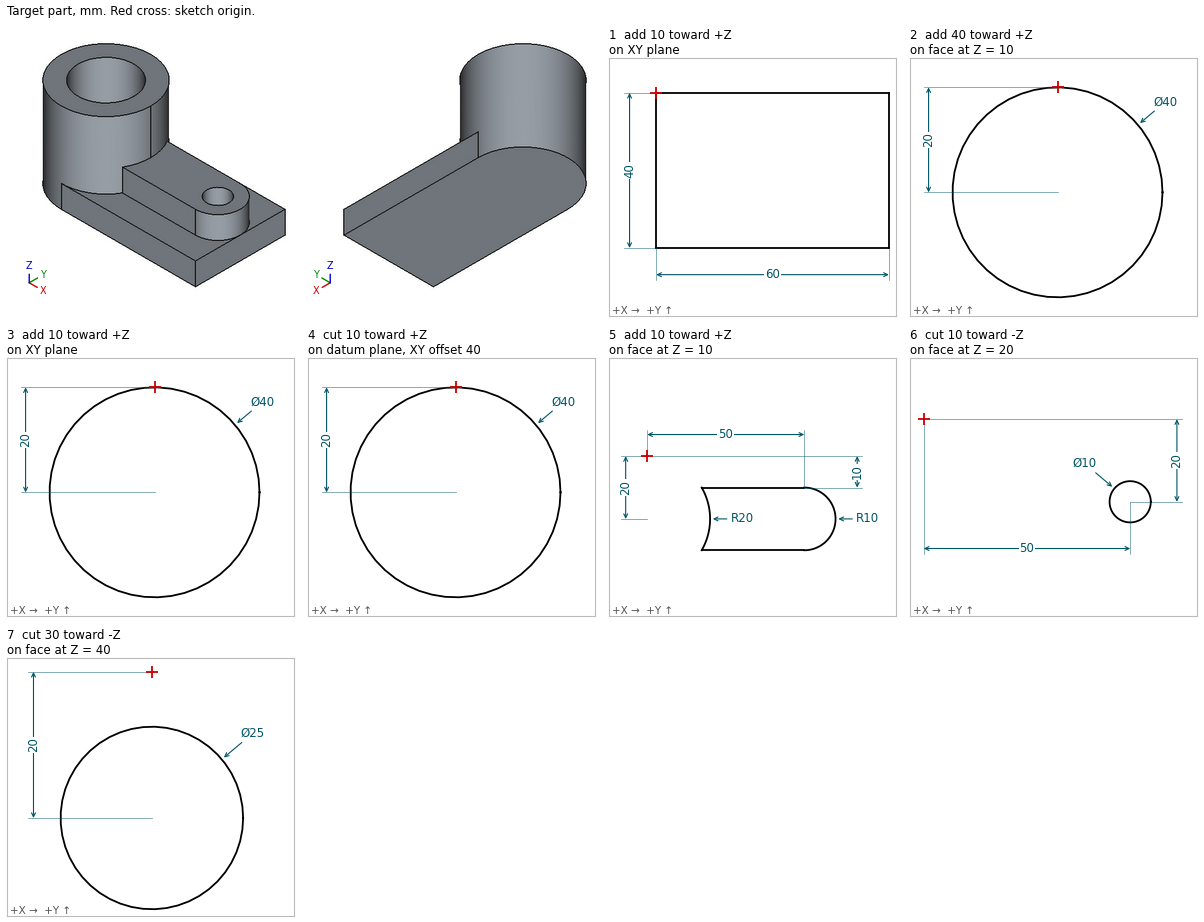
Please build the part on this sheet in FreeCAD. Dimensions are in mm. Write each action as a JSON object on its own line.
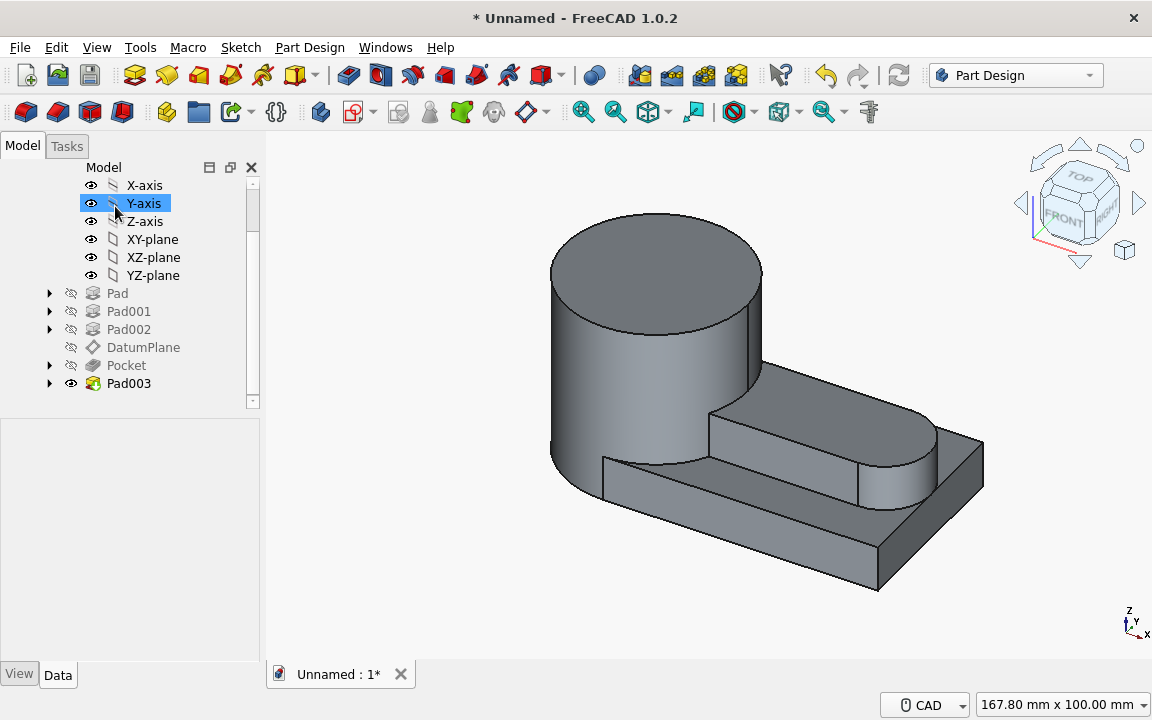
{"action": "left_click", "coordinate": [861, 428]}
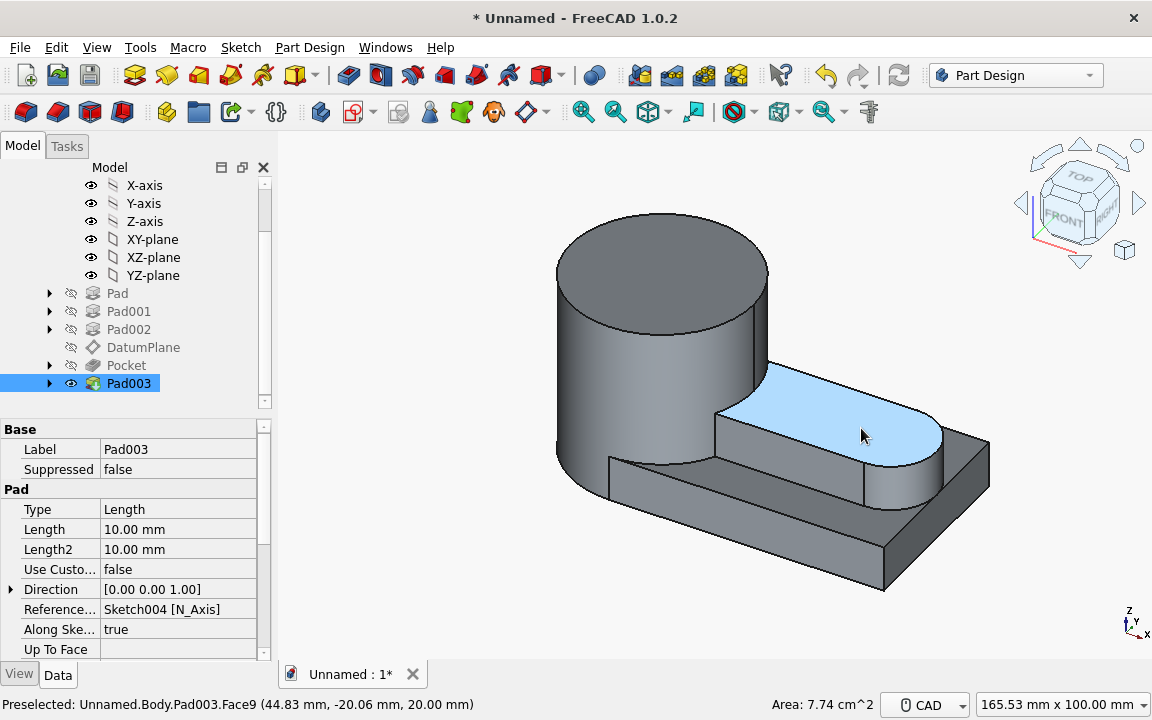
{"action": "left_click", "coordinate": [354, 112]}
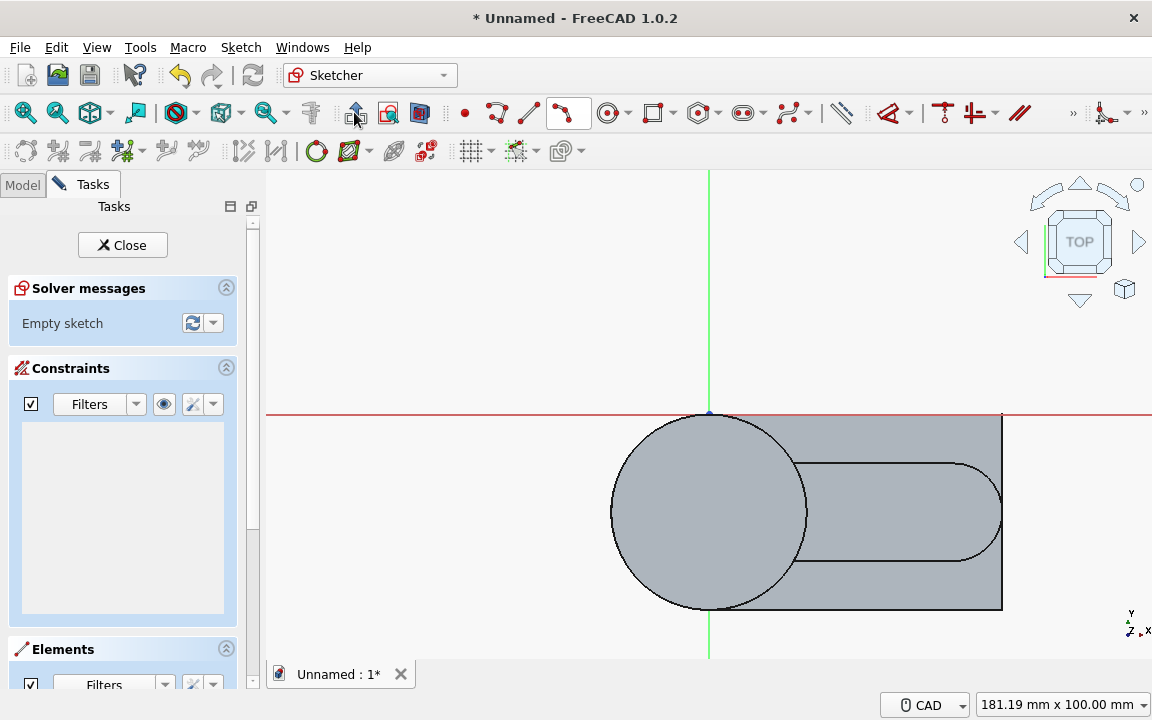
{"action": "left_click", "coordinate": [420, 114]}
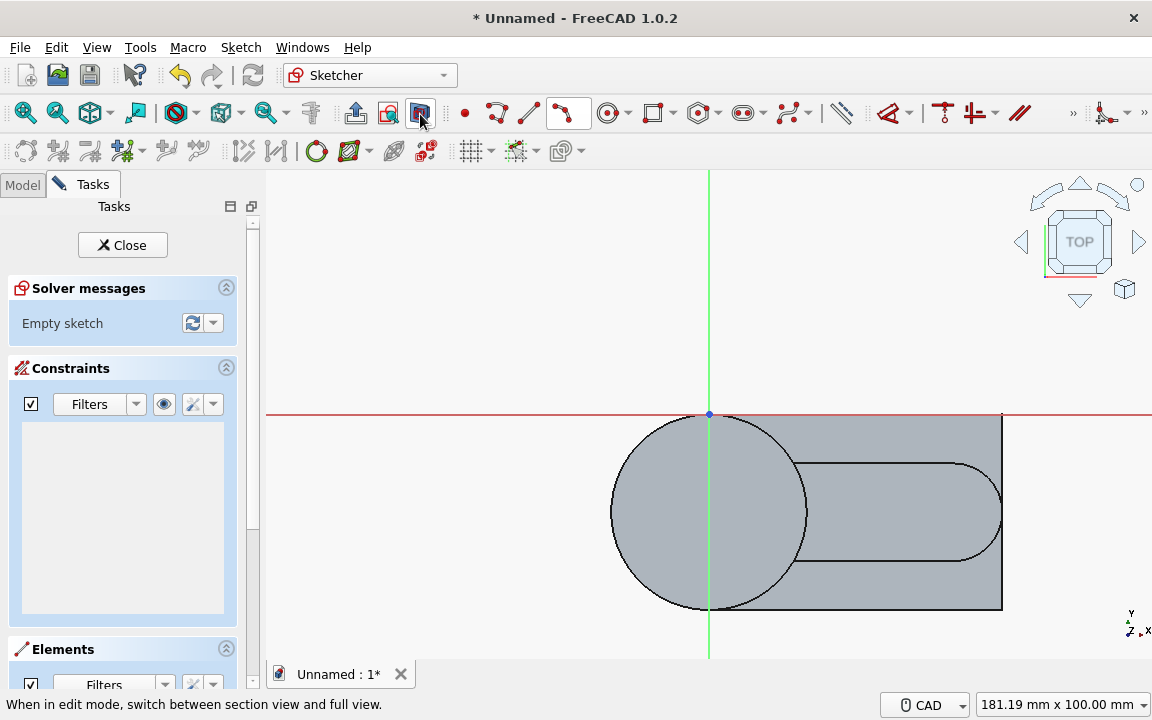
{"action": "scroll", "coordinate": [987, 532], "scroll_direction": "up", "scroll_amount": 9}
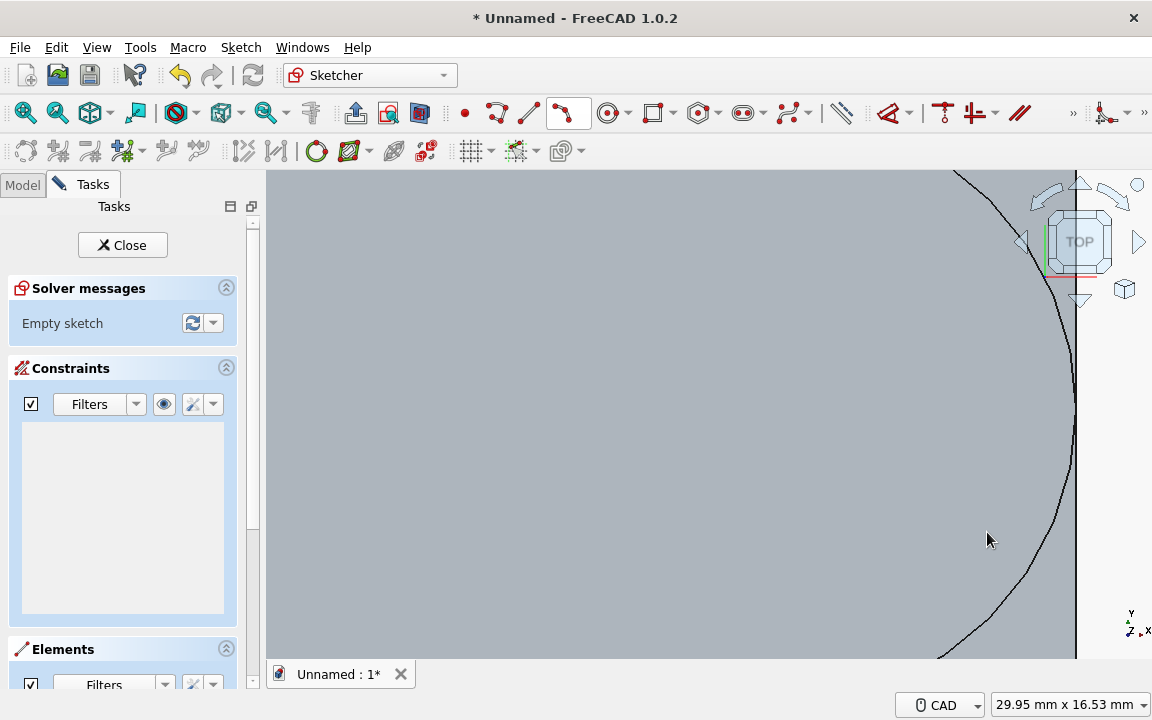
{"action": "left_click", "coordinate": [608, 114]}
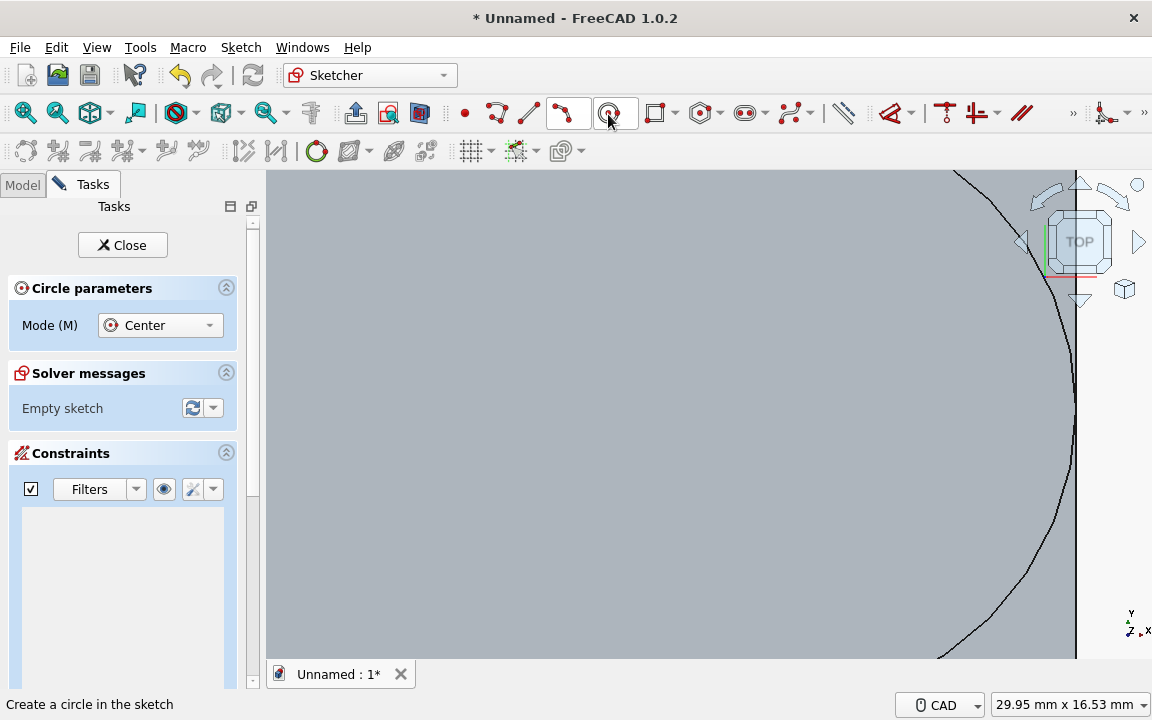
{"action": "left_click", "coordinate": [780, 409]}
{"action": "left_click", "coordinate": [885, 304]}
{"action": "key", "text": "Escape"}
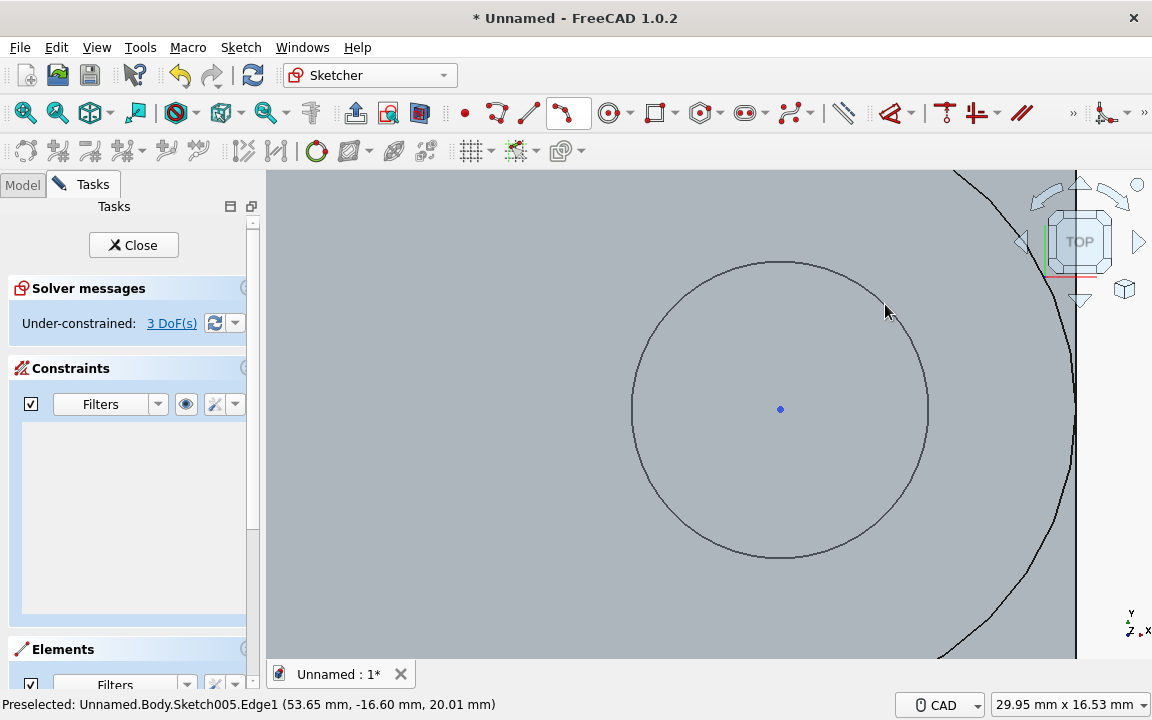
{"action": "left_click", "coordinate": [890, 114]}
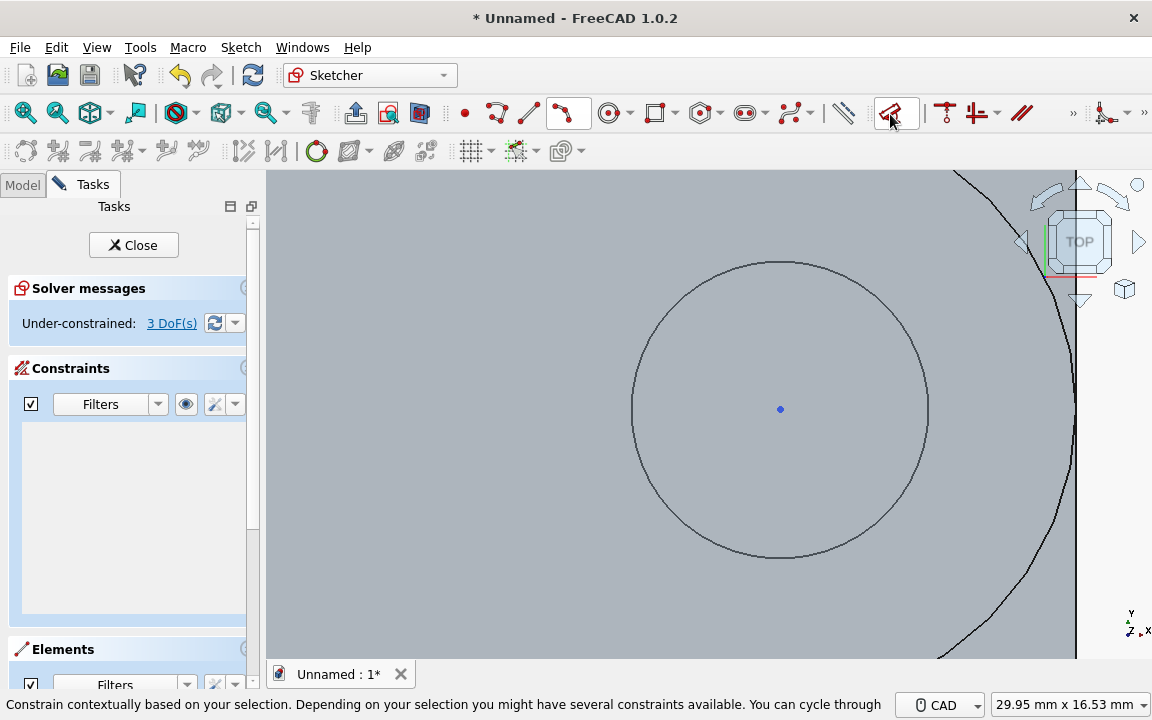
{"action": "left_click", "coordinate": [885, 305]}
{"action": "left_click", "coordinate": [908, 282]}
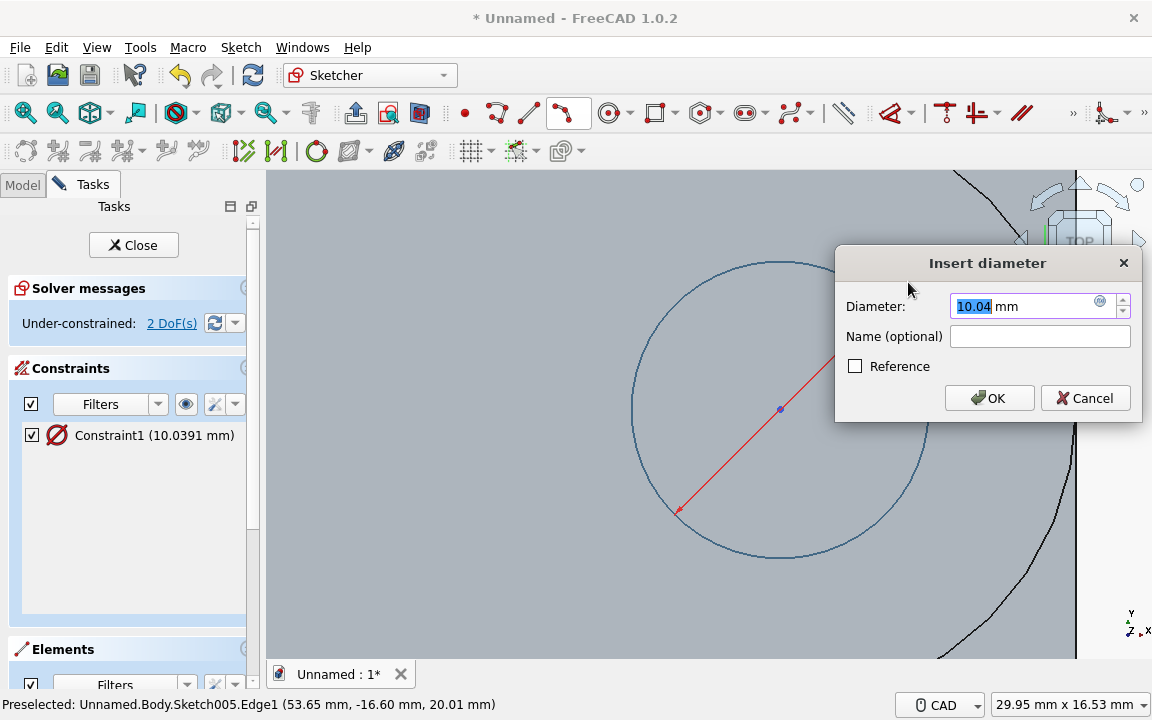
{"action": "type", "text": "10"}
{"action": "key", "text": "Return"}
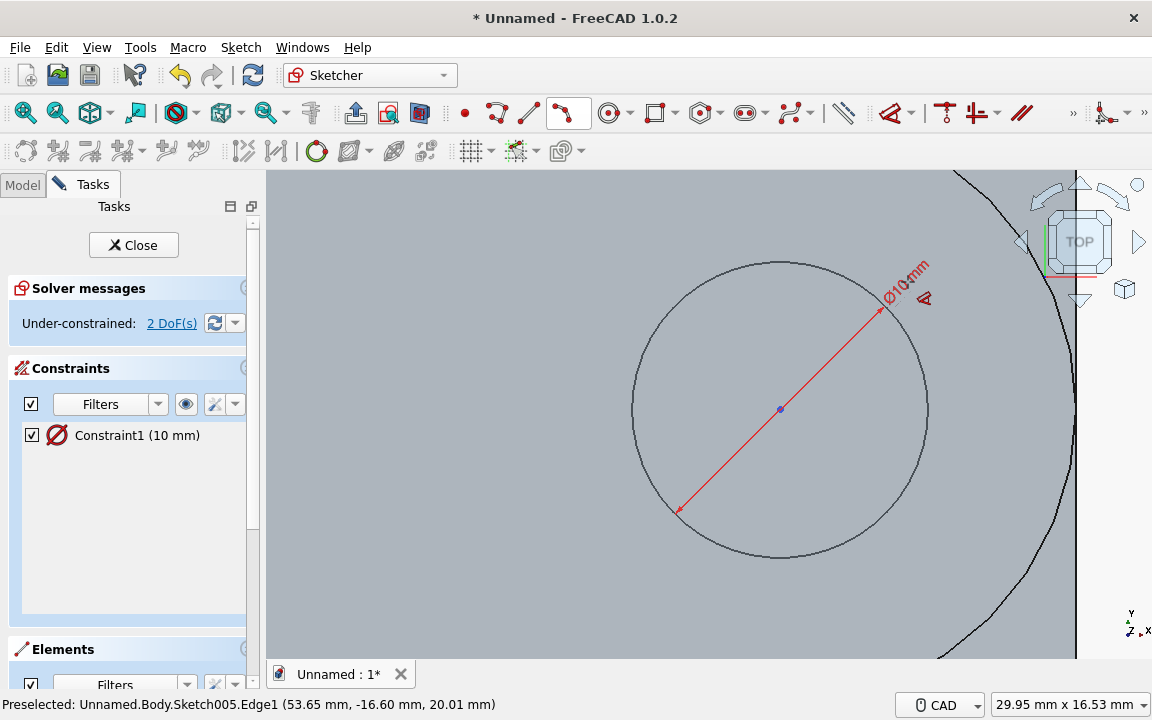
{"action": "left_click", "coordinate": [780, 410]}
{"action": "left_click", "coordinate": [537, 444]}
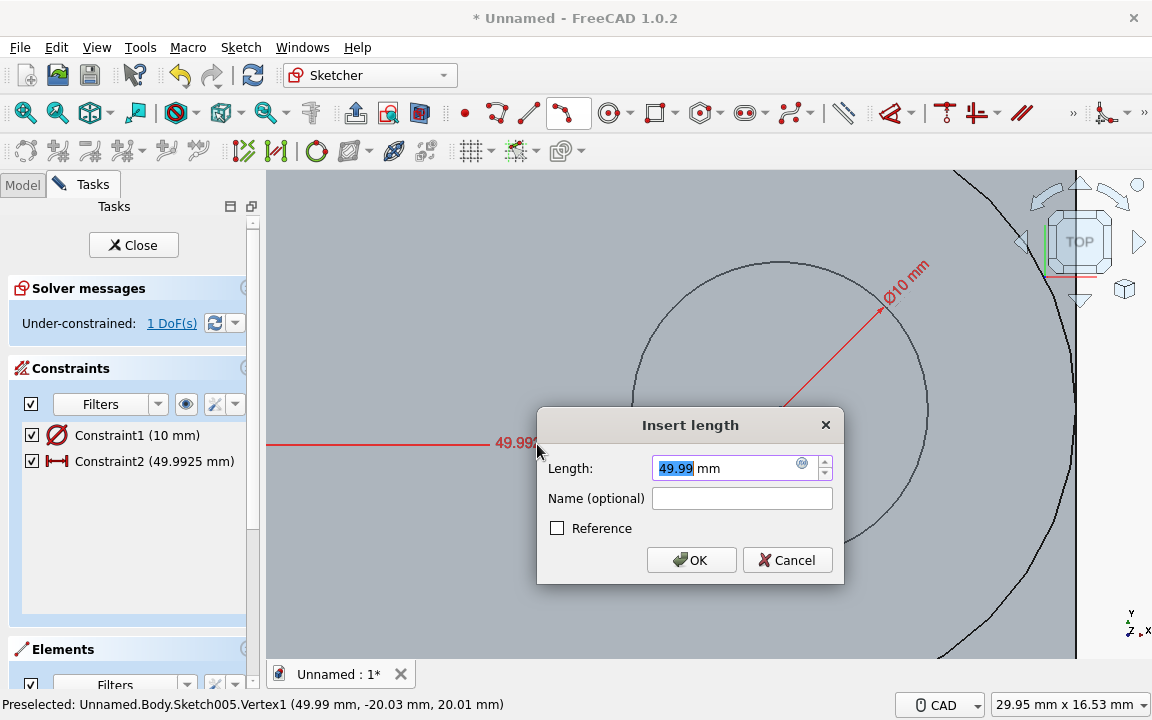
{"action": "type", "text": "50"}
{"action": "key", "text": "Return"}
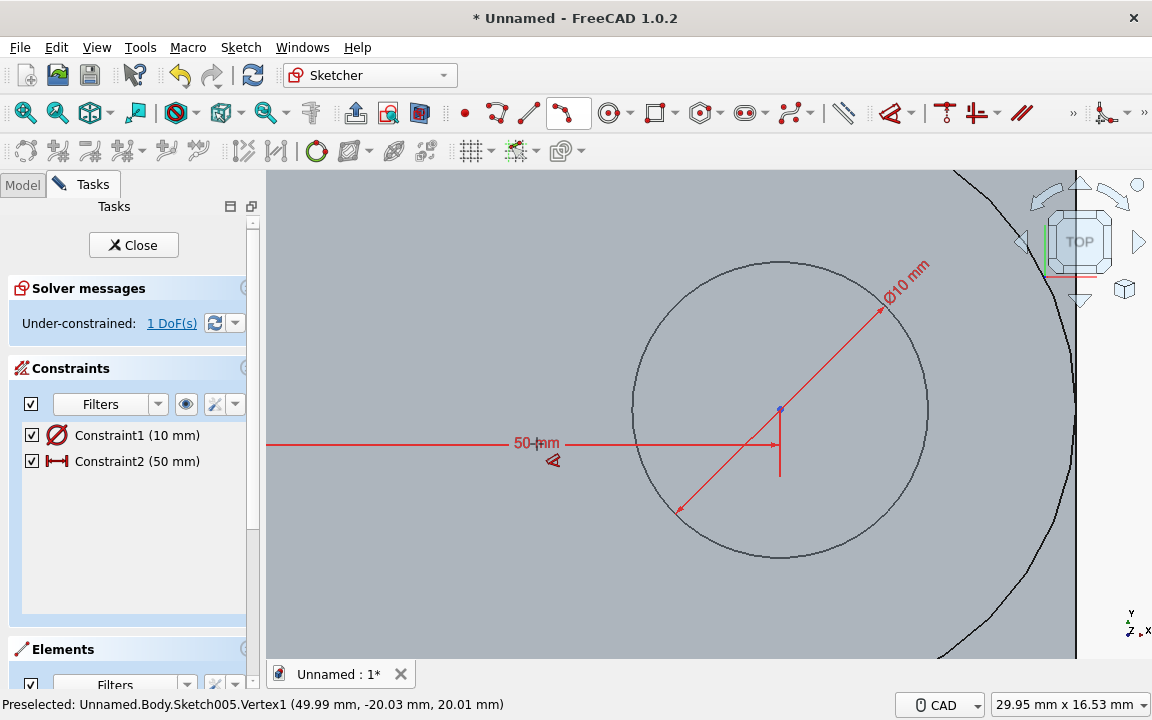
{"action": "left_click", "coordinate": [780, 410]}
{"action": "left_click", "coordinate": [814, 304]}